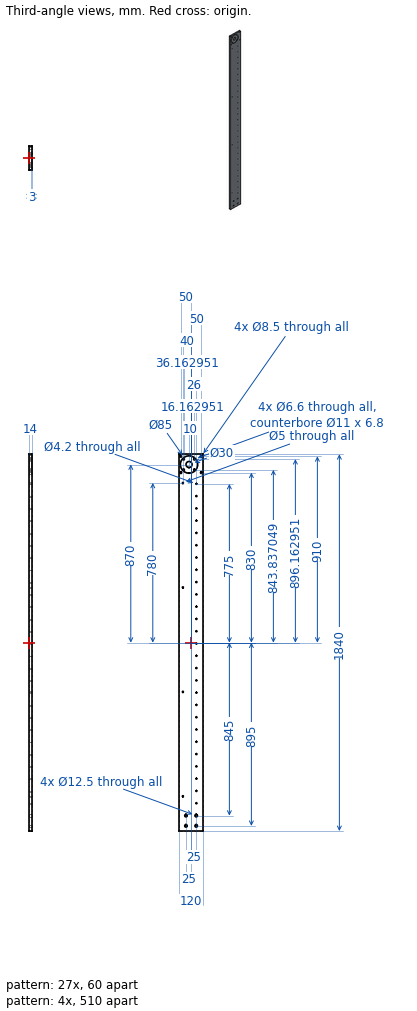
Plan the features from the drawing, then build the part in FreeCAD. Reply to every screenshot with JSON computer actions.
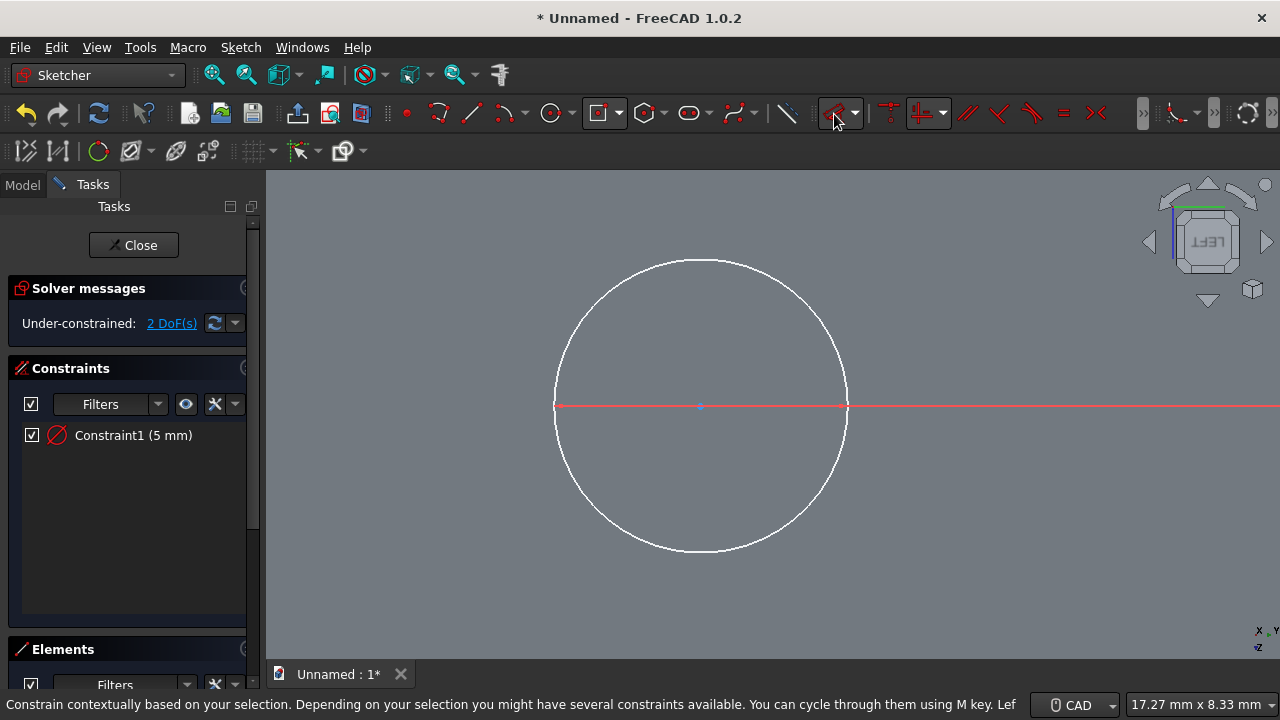
{"action": "left_click", "coordinate": [701, 406]}
{"action": "left_click", "coordinate": [908, 440]}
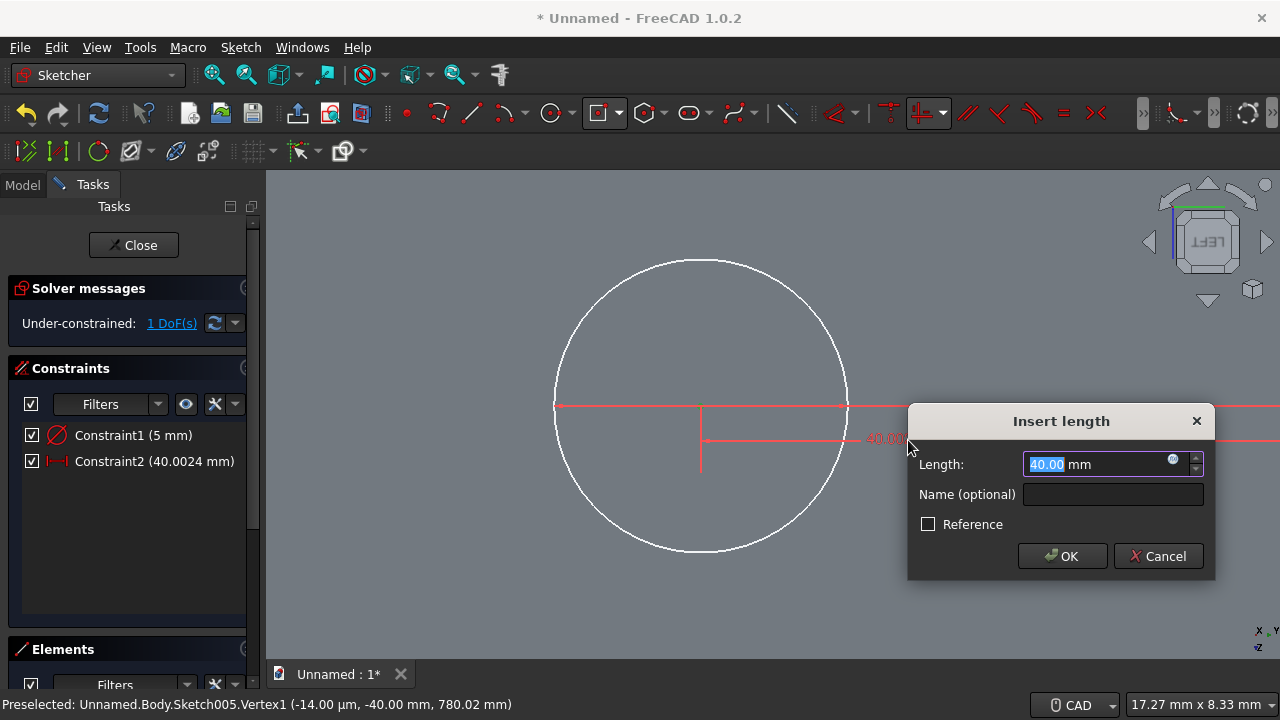
{"action": "type", "text": "40"}
{"action": "key", "text": "Return"}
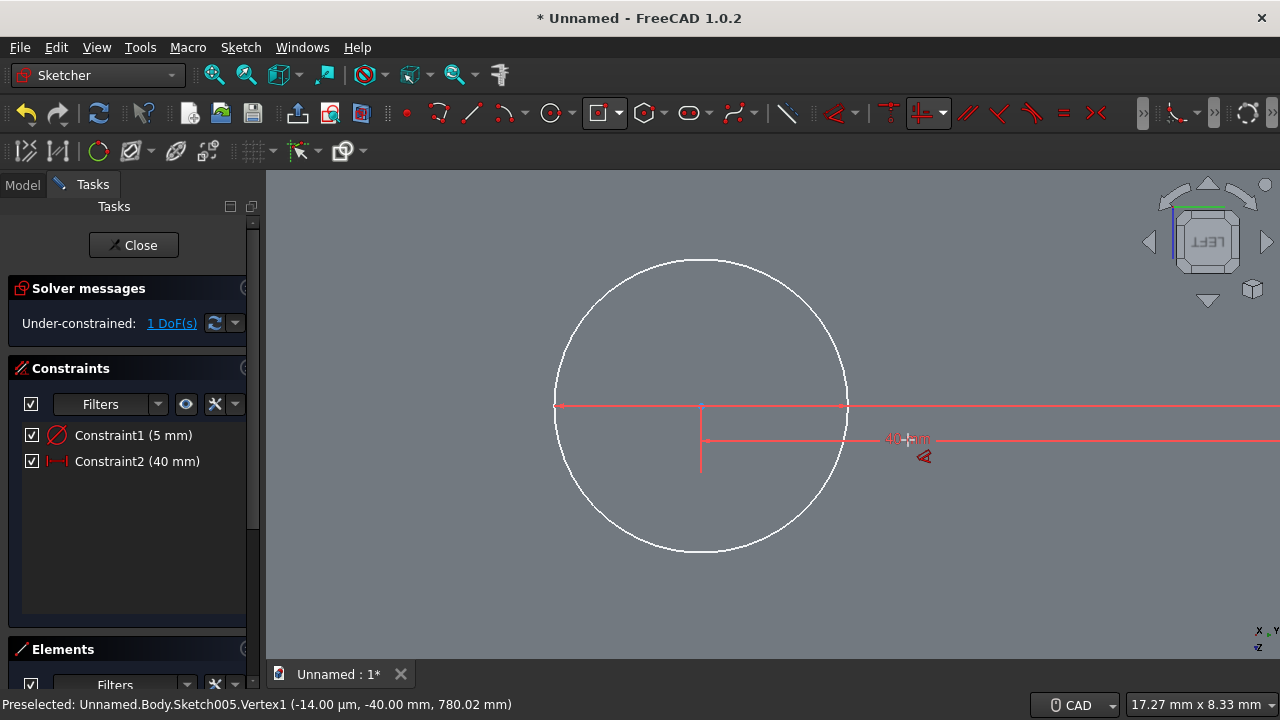
{"action": "left_click", "coordinate": [701, 406]}
{"action": "left_click", "coordinate": [667, 302]}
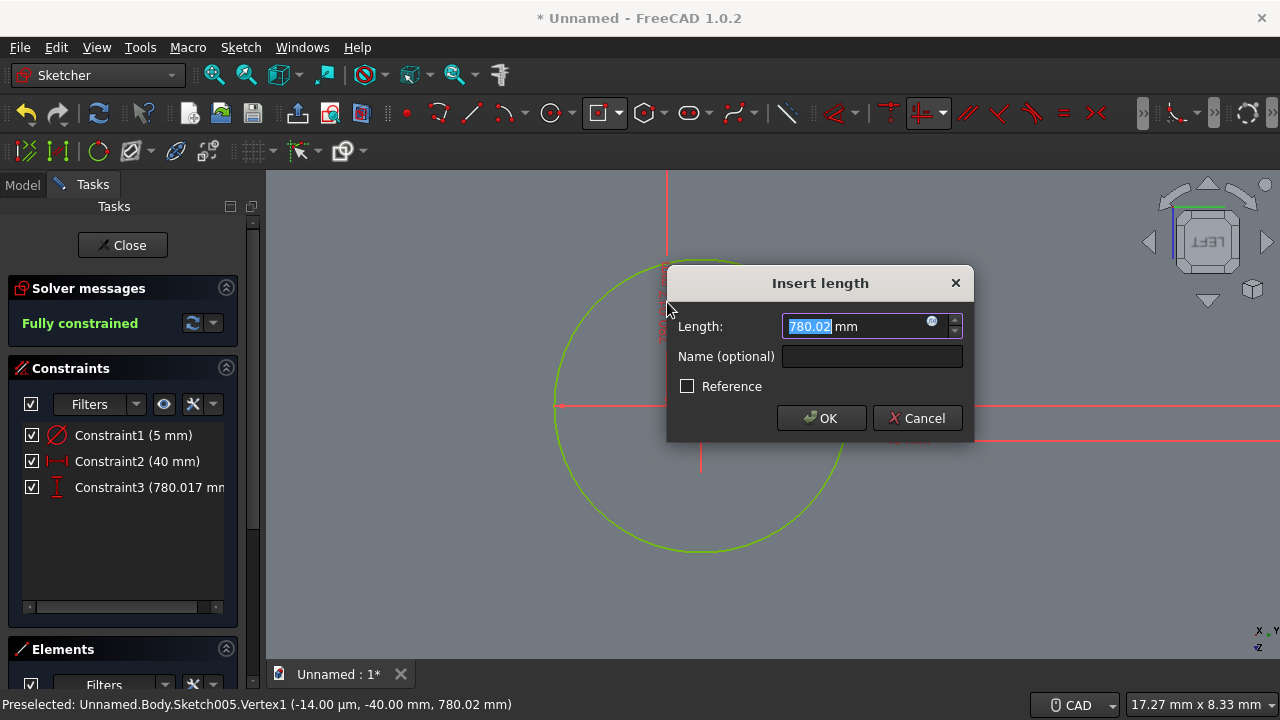
{"action": "type", "text": "780"}
{"action": "key", "text": "Return"}
{"action": "key", "text": "Escape"}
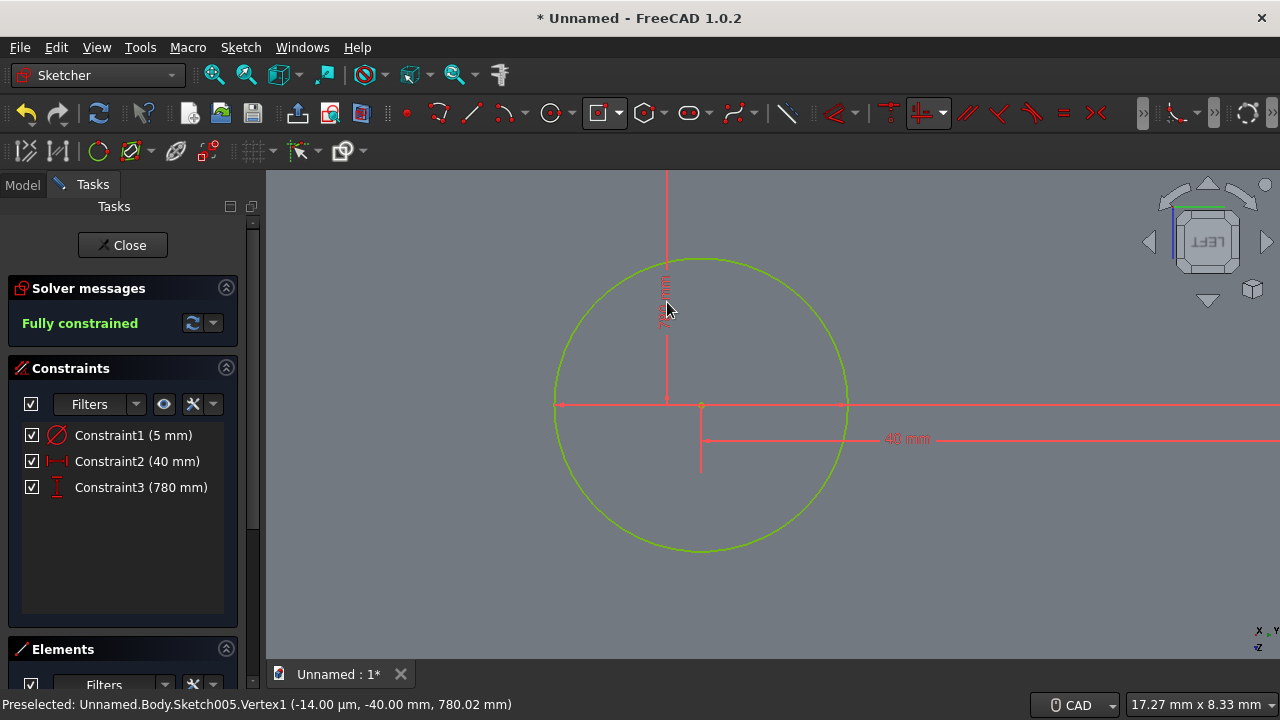
{"action": "left_click", "coordinate": [123, 245]}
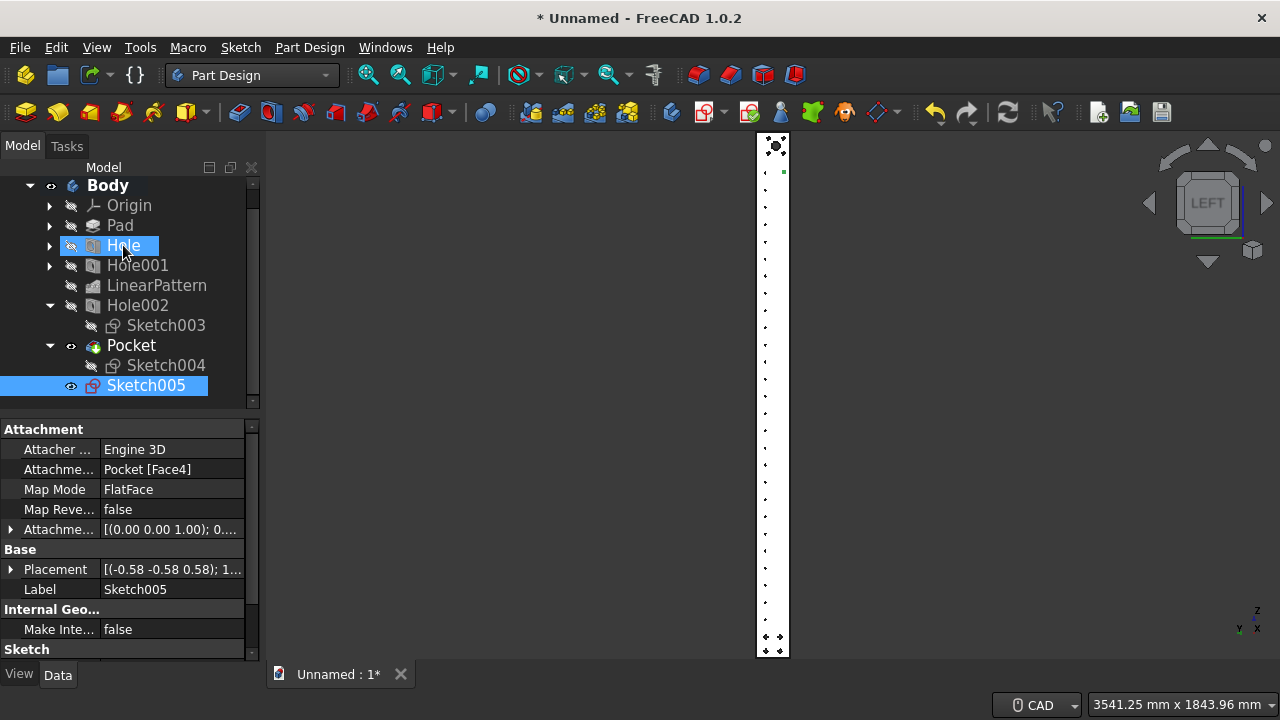
{"action": "left_click", "coordinate": [272, 112]}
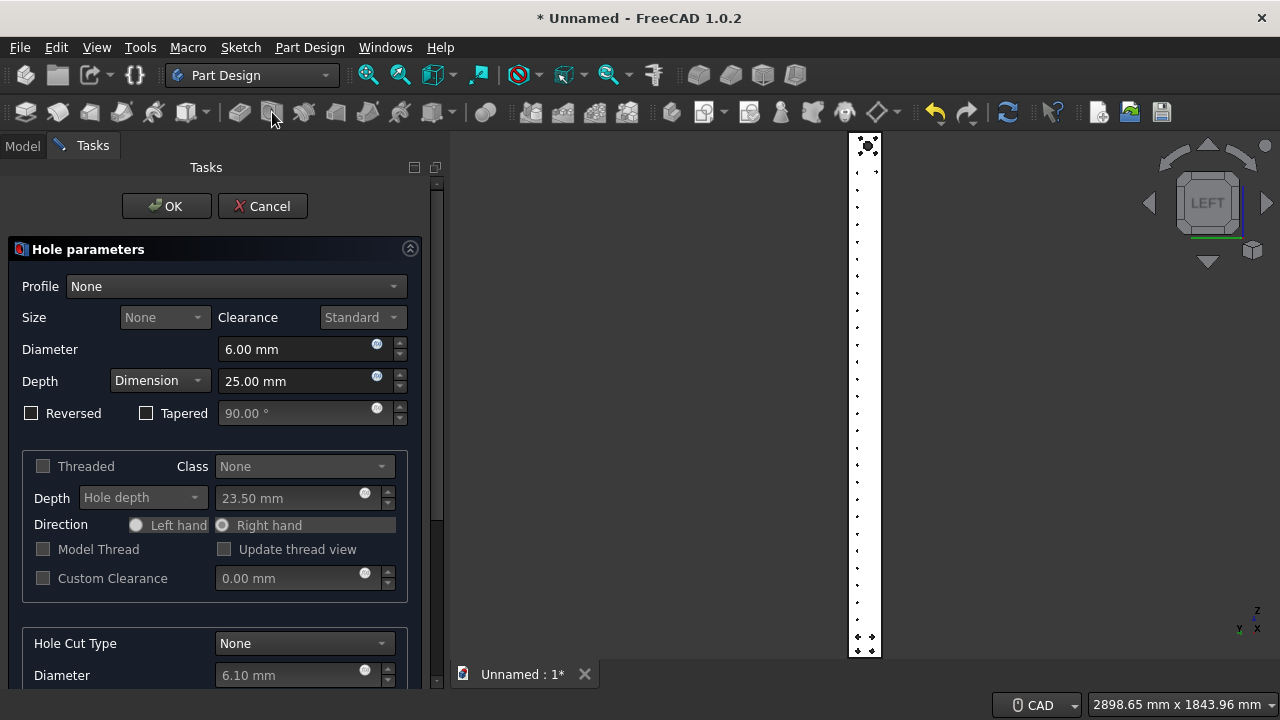
{"action": "triple_click", "coordinate": [305, 349]}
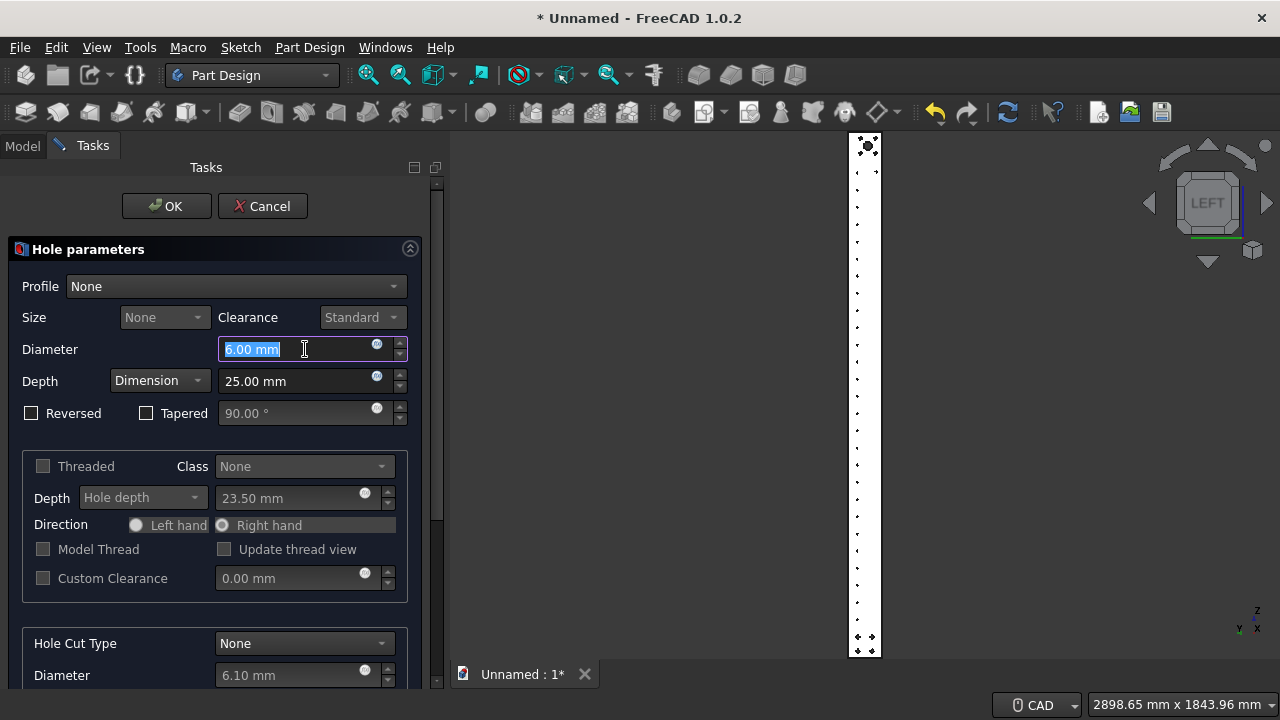
{"action": "type", "text": "5"}
{"action": "key", "text": "Tab"}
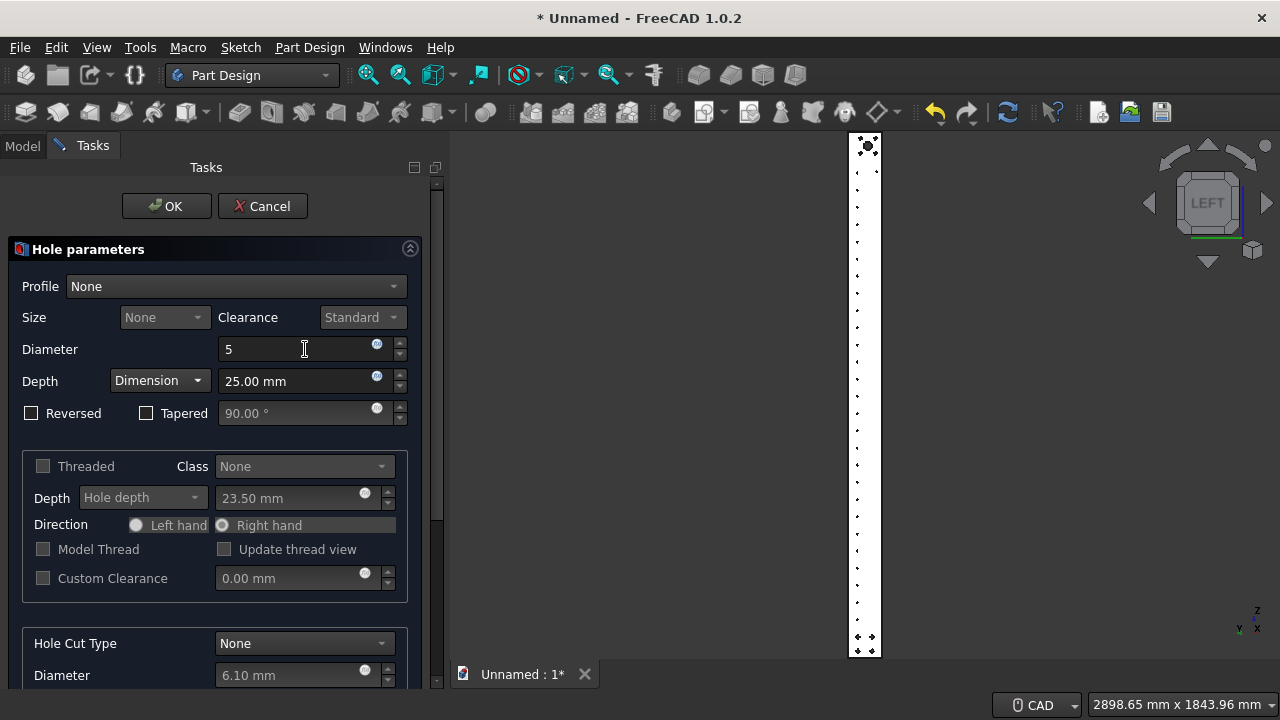
{"action": "left_click", "coordinate": [161, 380]}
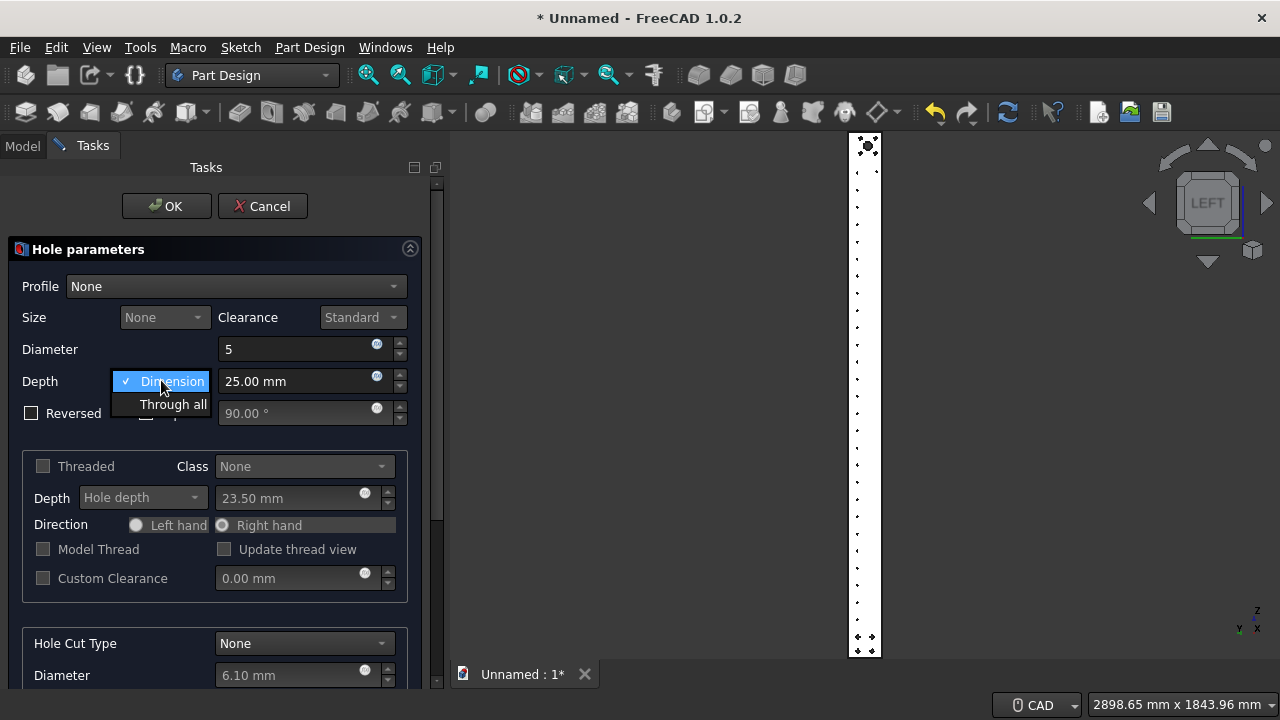
{"action": "left_click", "coordinate": [160, 404]}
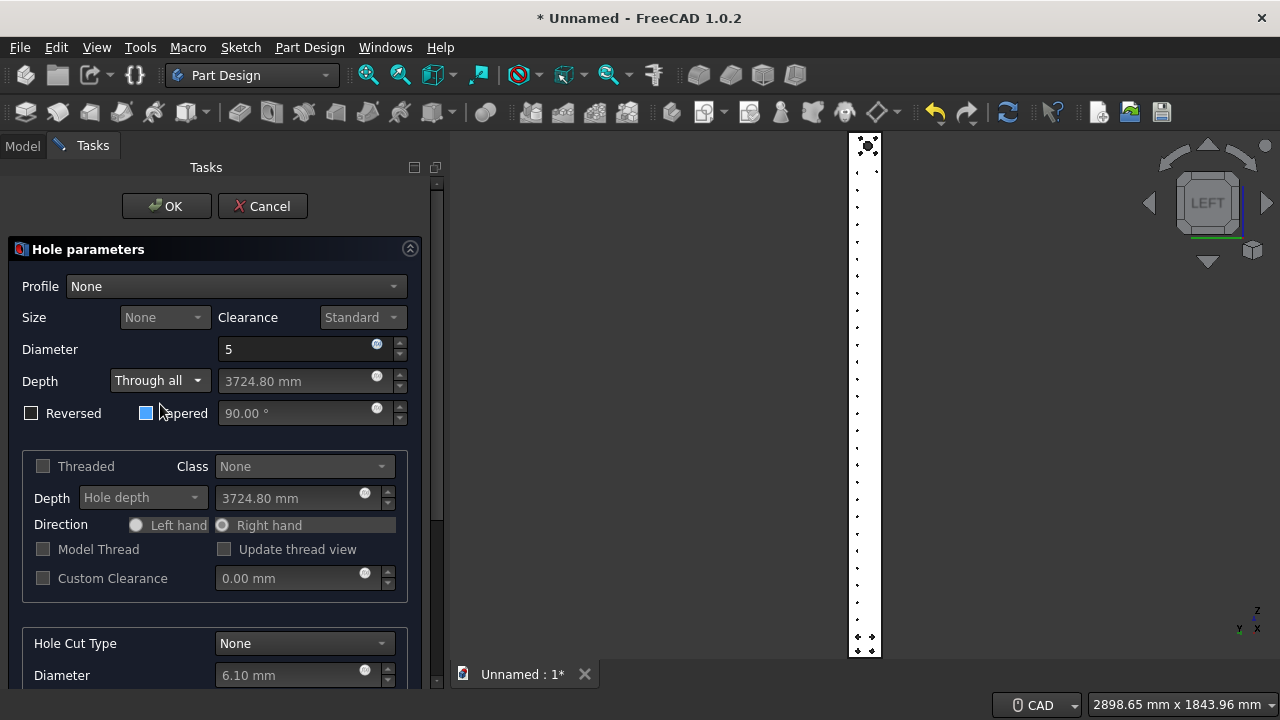
{"action": "left_click", "coordinate": [167, 206]}